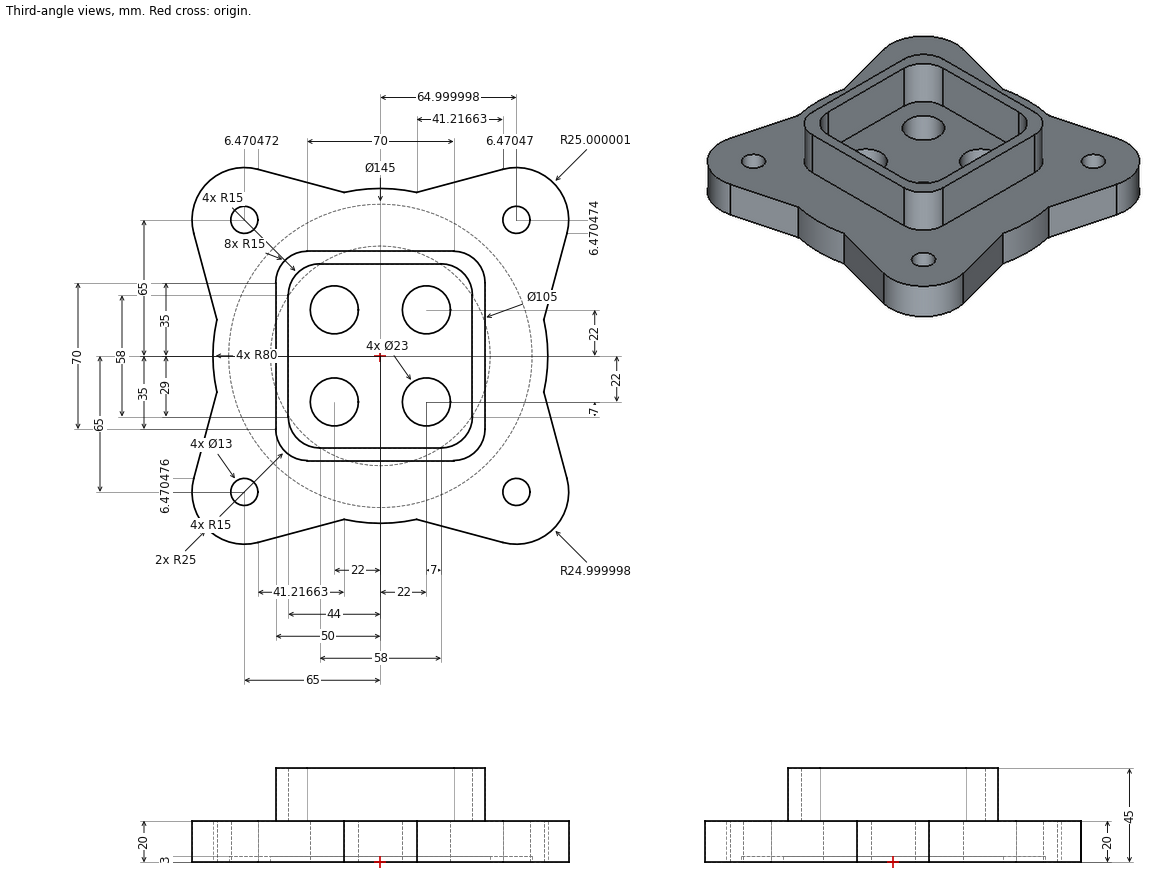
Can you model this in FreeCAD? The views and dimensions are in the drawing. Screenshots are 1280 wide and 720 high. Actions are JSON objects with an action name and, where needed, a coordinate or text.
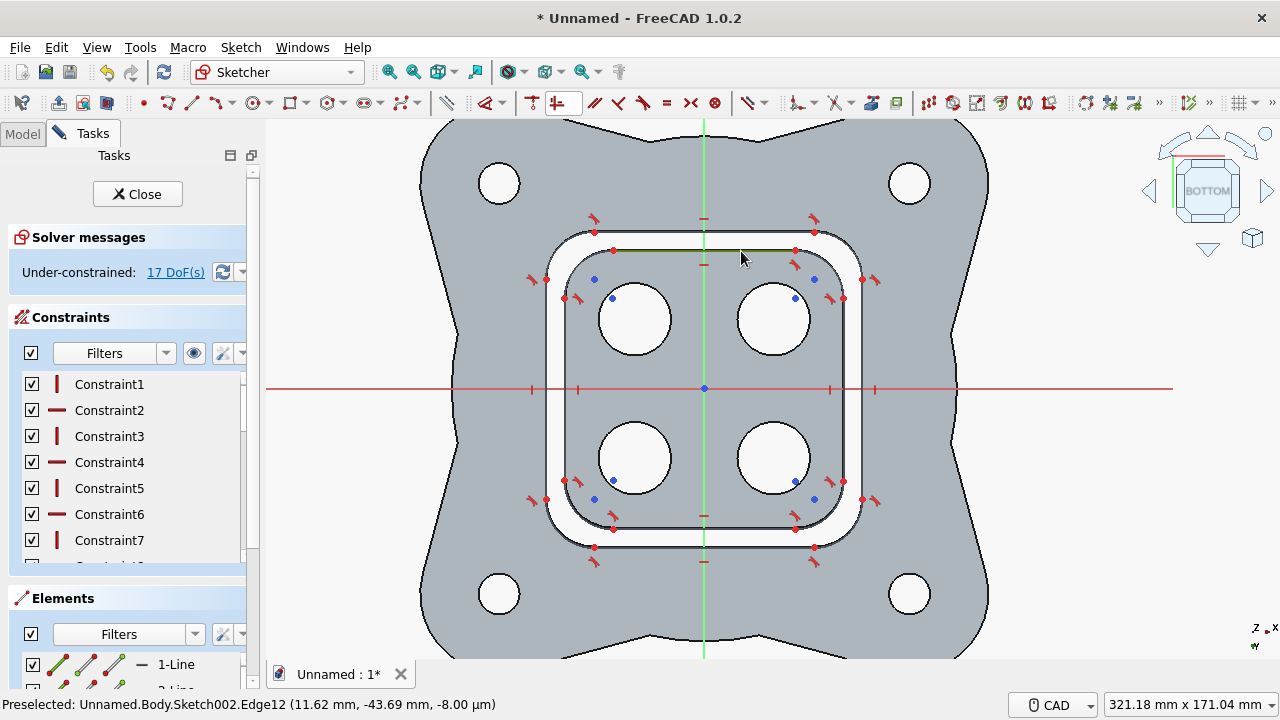
{"action": "left_click", "coordinate": [591, 256]}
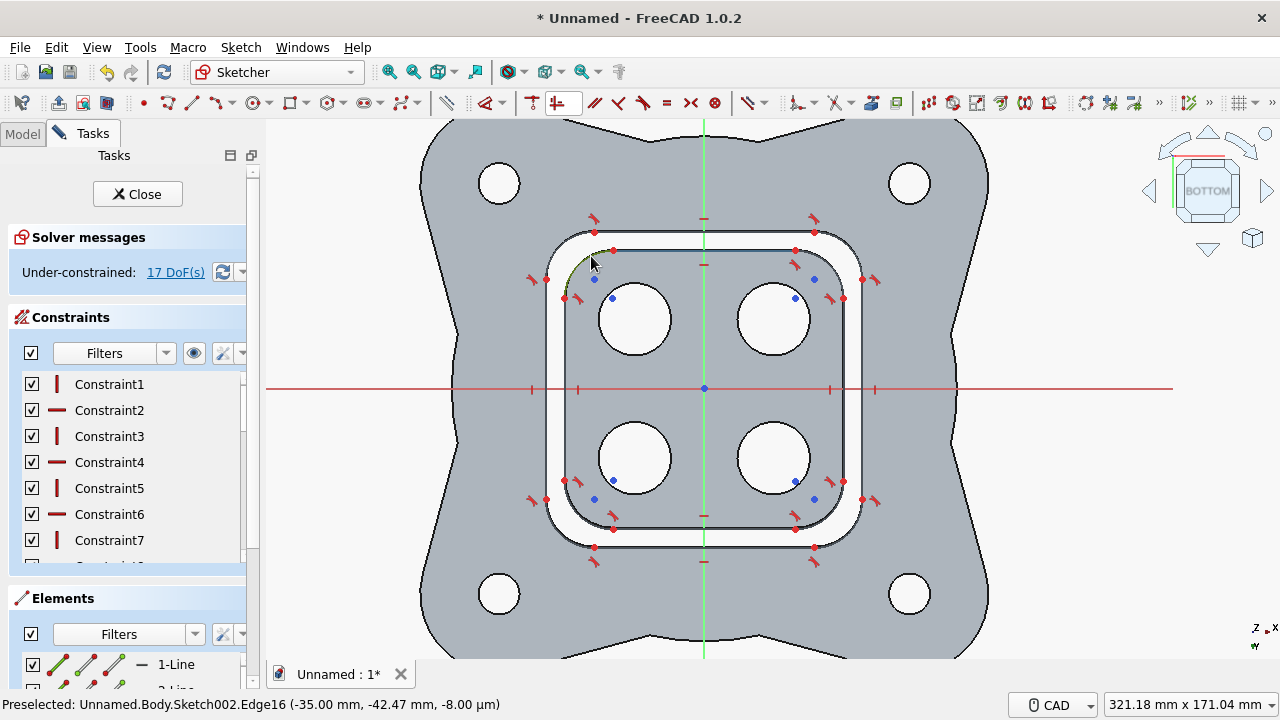
{"action": "key", "text": "t"}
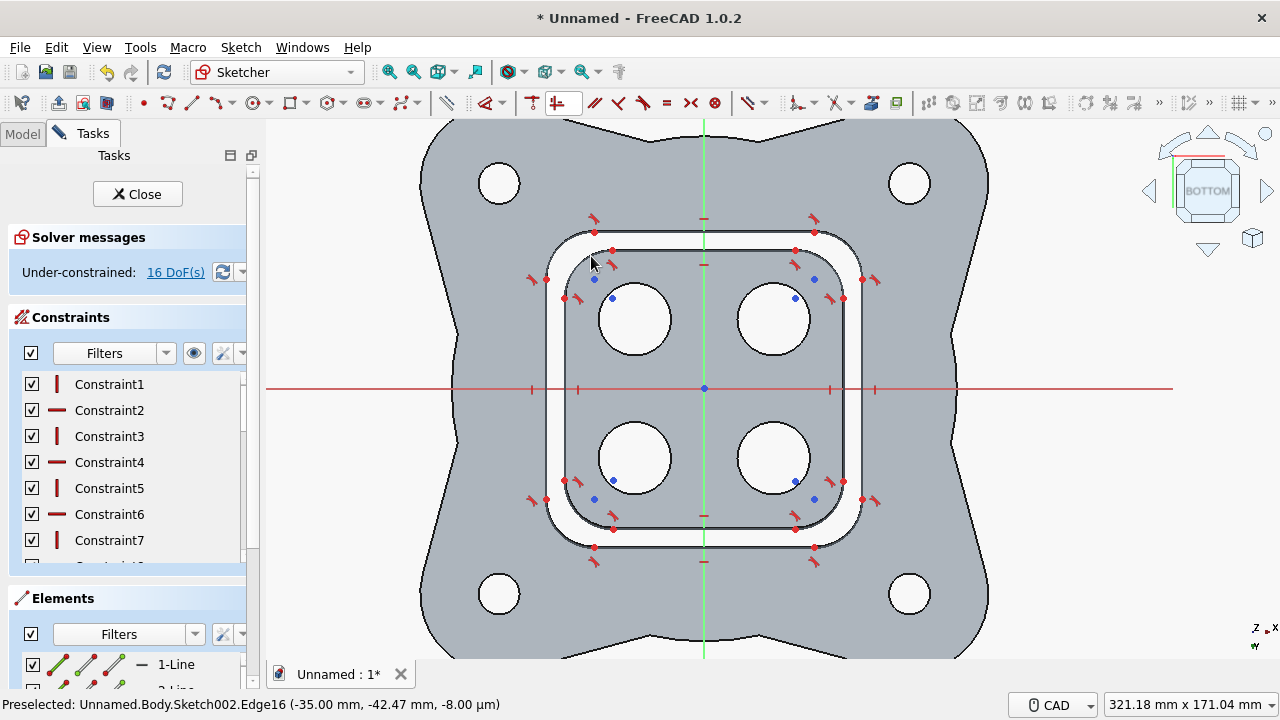
{"action": "left_click", "coordinate": [572, 237]}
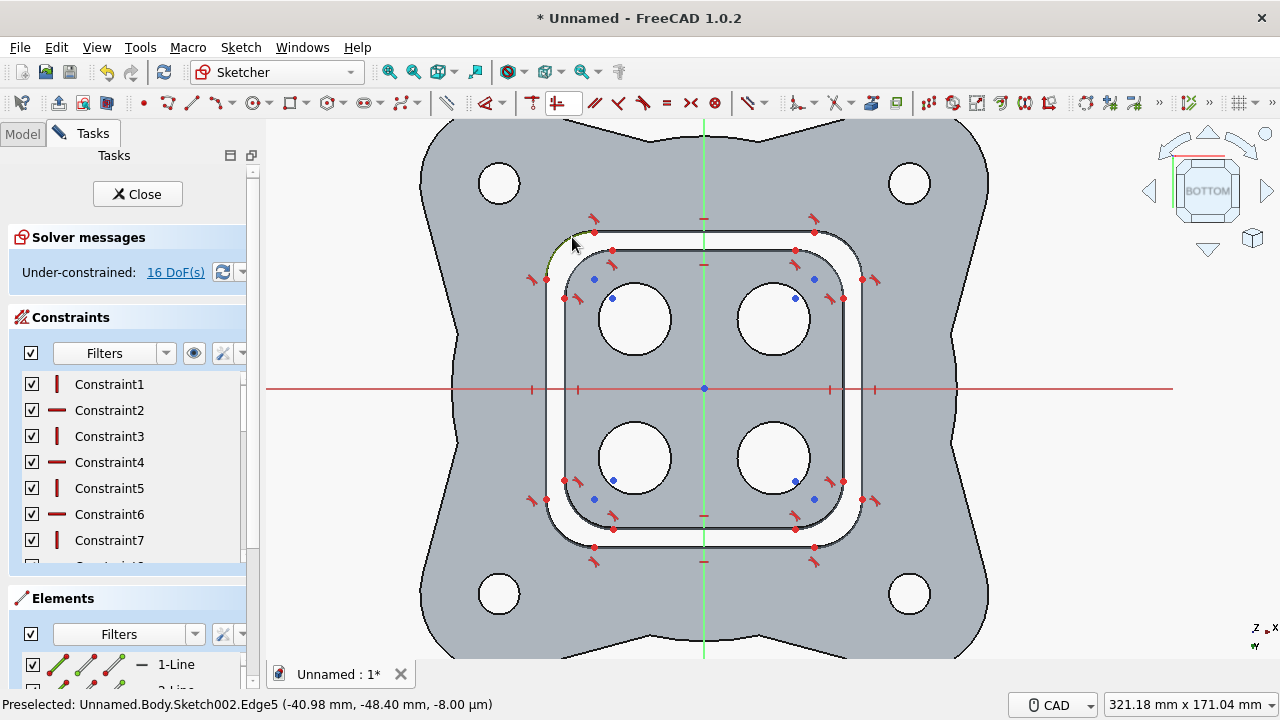
{"action": "left_click", "coordinate": [857, 258]}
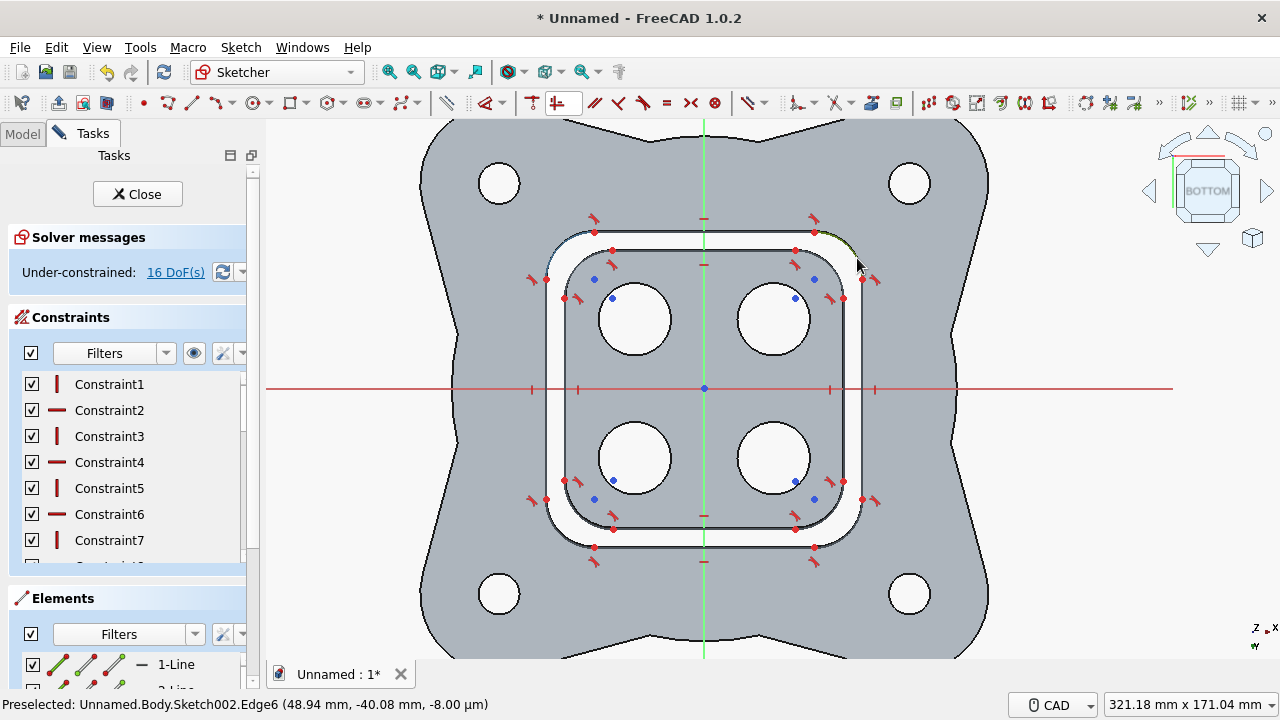
{"action": "left_click", "coordinate": [836, 543]}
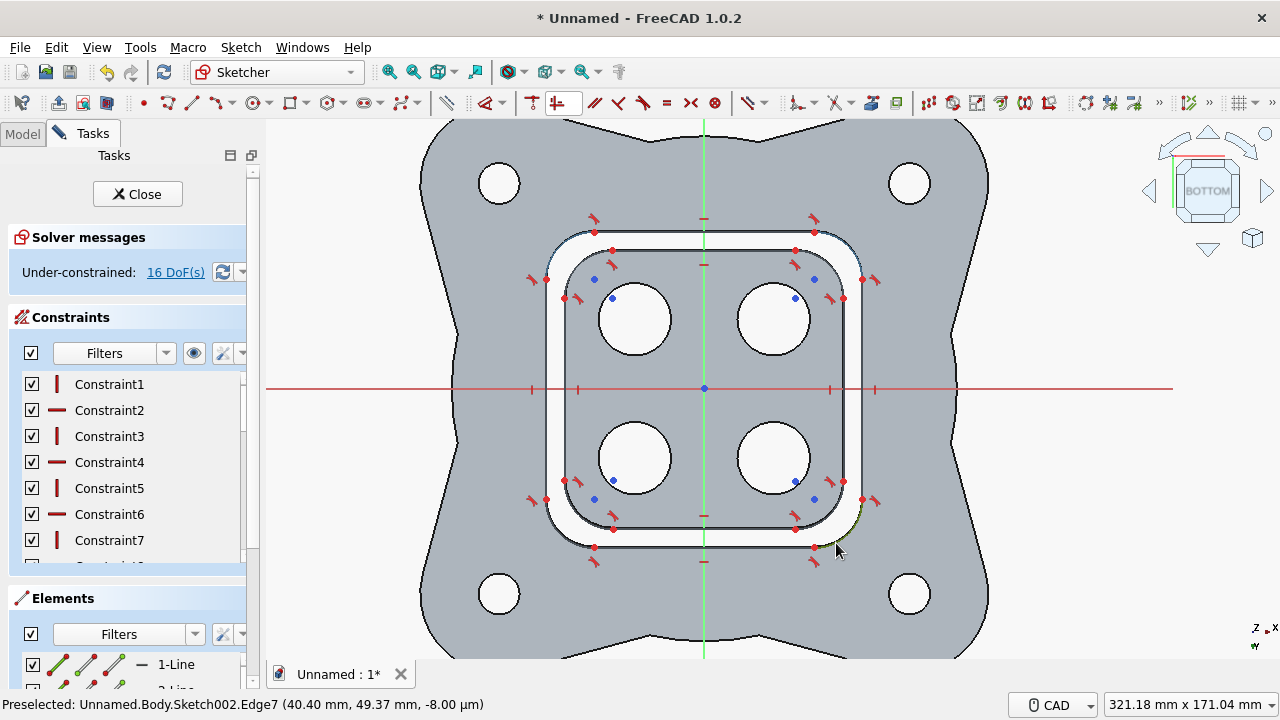
{"action": "left_click", "coordinate": [551, 522]}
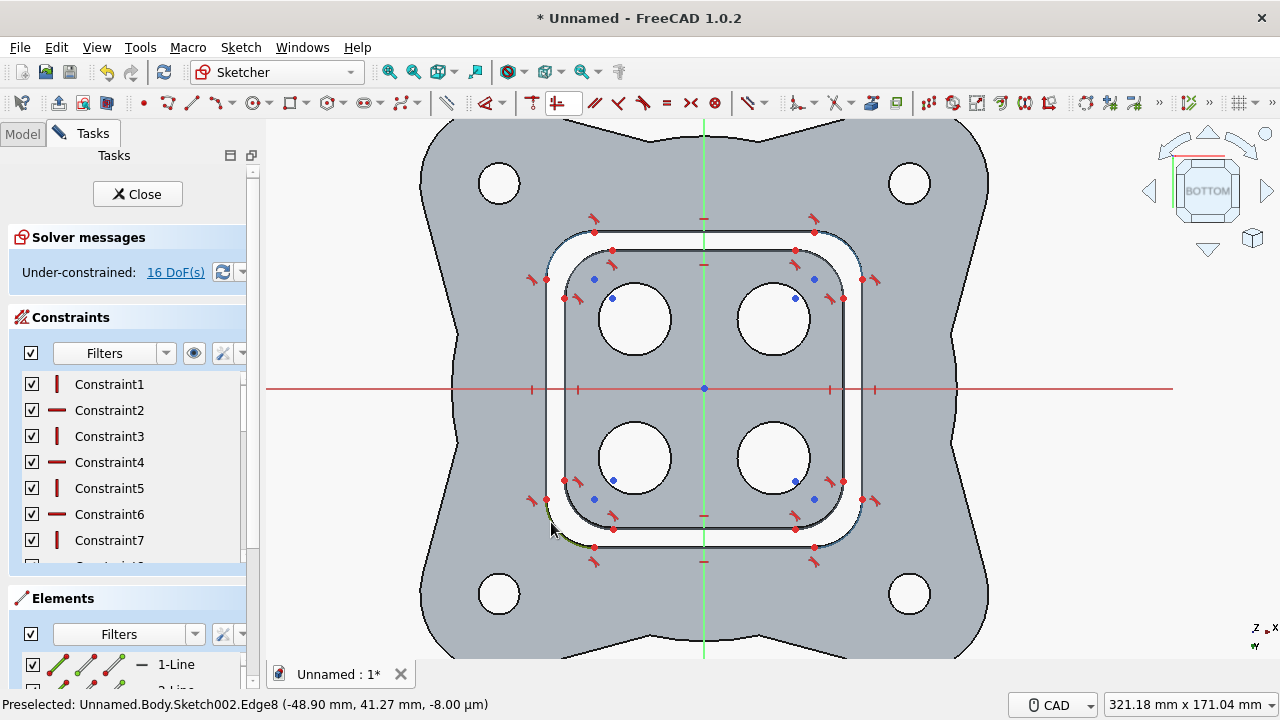
{"action": "left_click", "coordinate": [570, 503]}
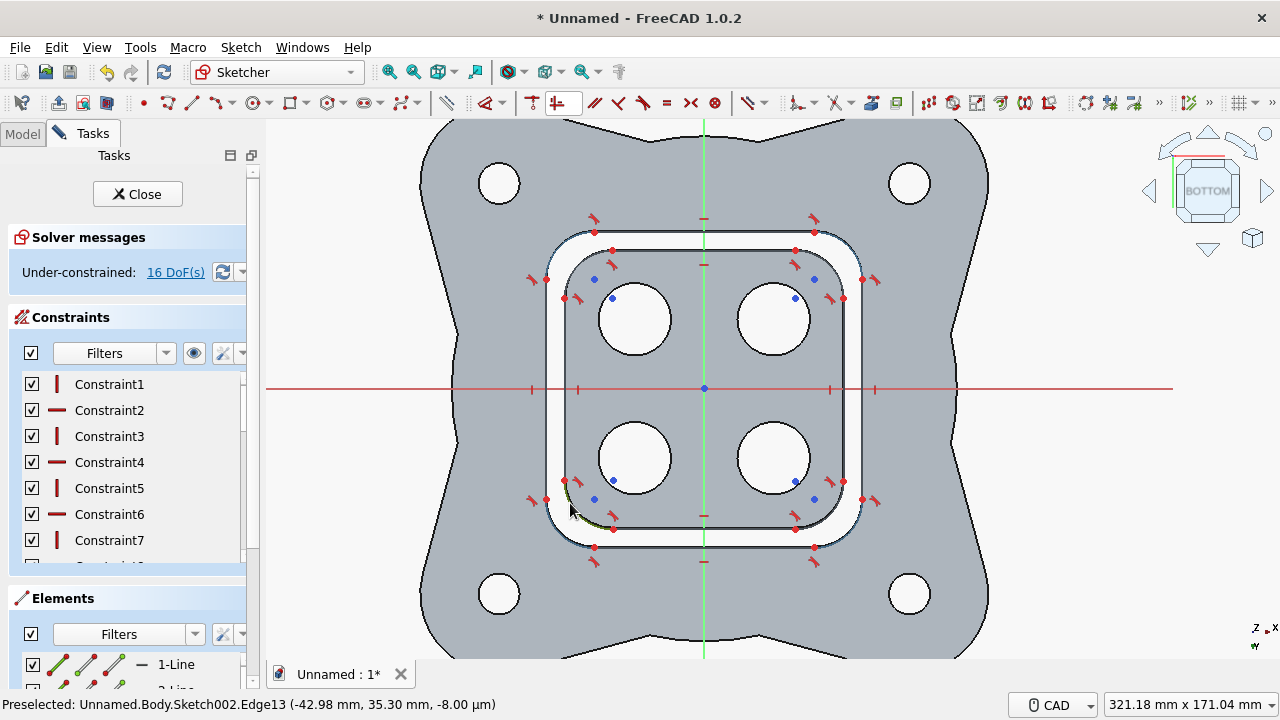
{"action": "left_click", "coordinate": [817, 524]}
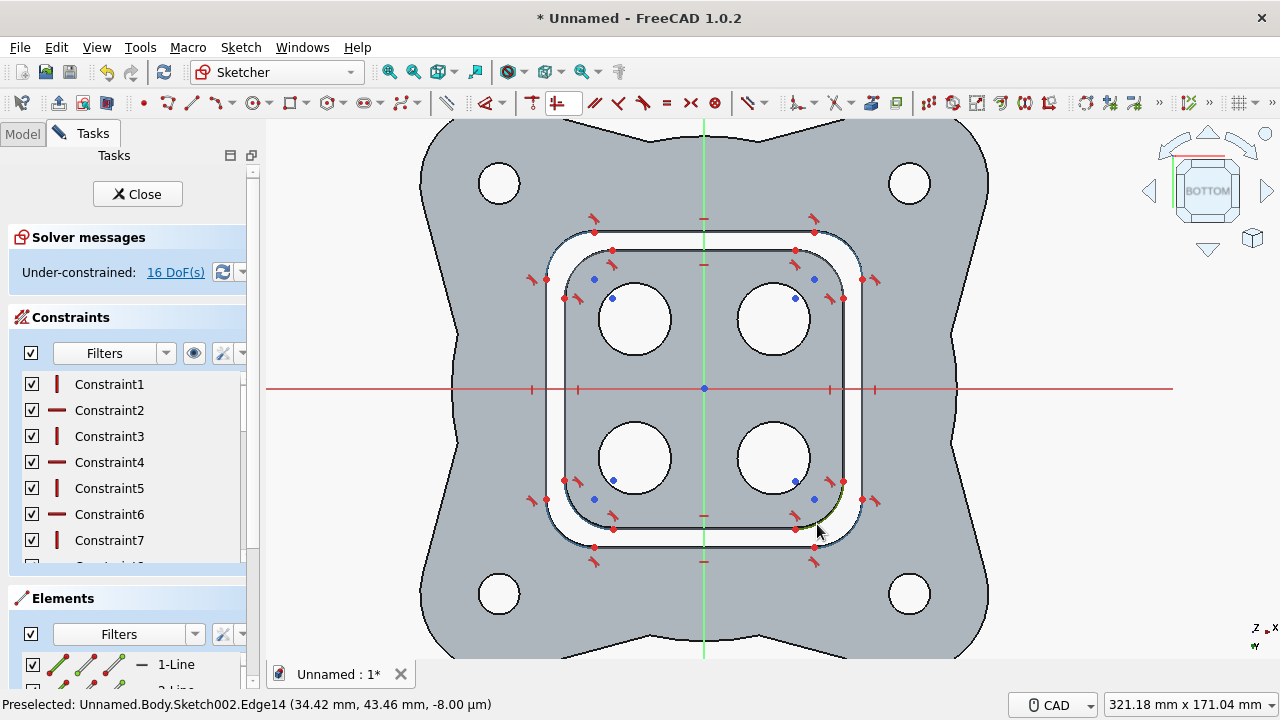
{"action": "left_click", "coordinate": [838, 277]}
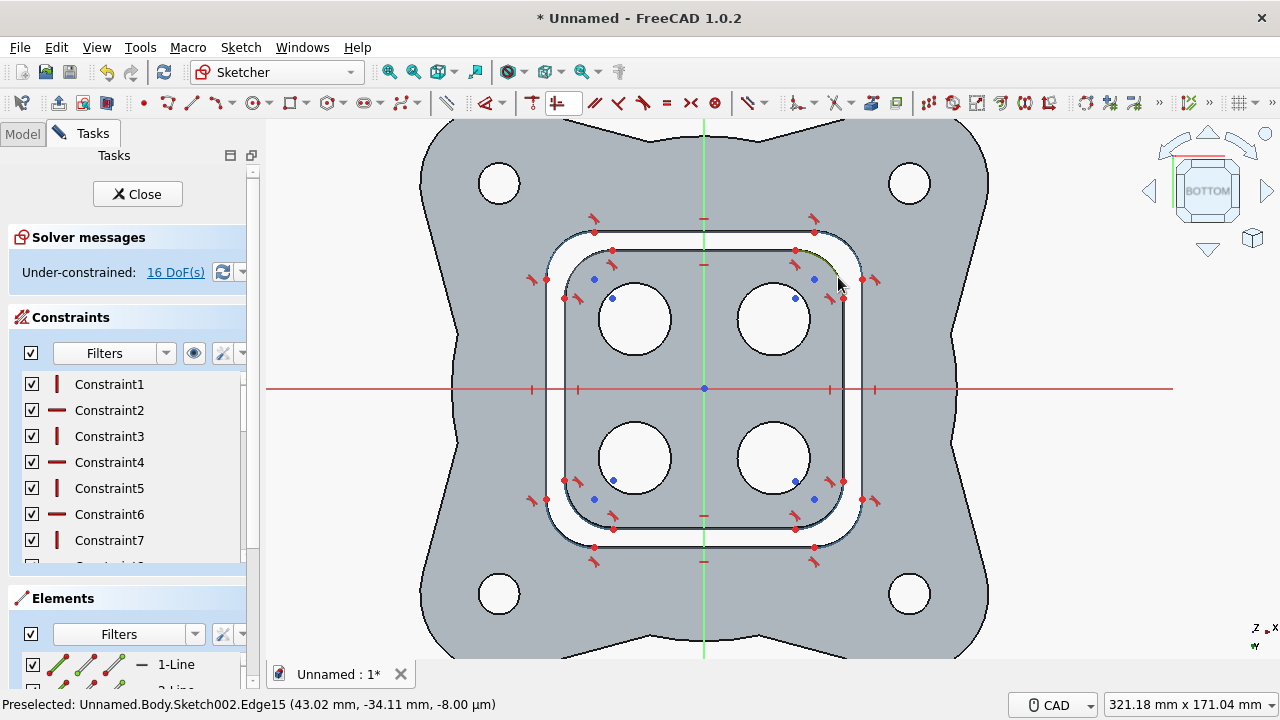
{"action": "left_click", "coordinate": [591, 256]}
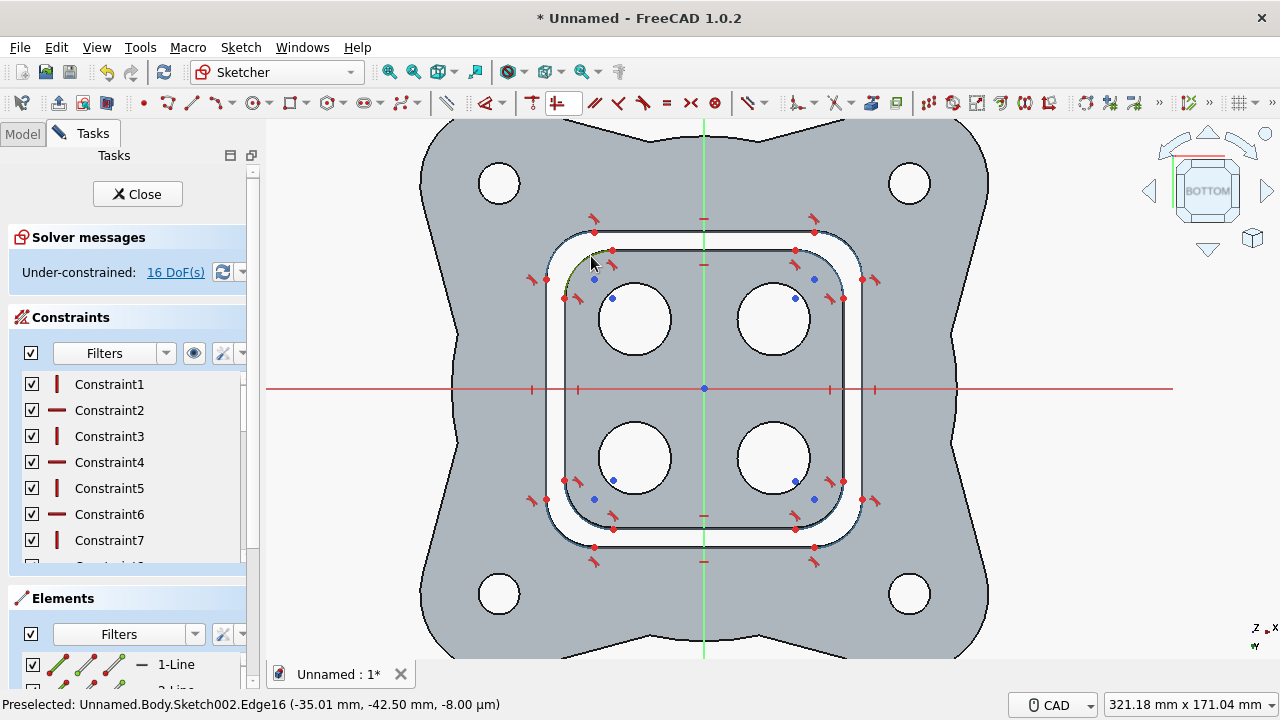
{"action": "left_click", "coordinate": [668, 104]}